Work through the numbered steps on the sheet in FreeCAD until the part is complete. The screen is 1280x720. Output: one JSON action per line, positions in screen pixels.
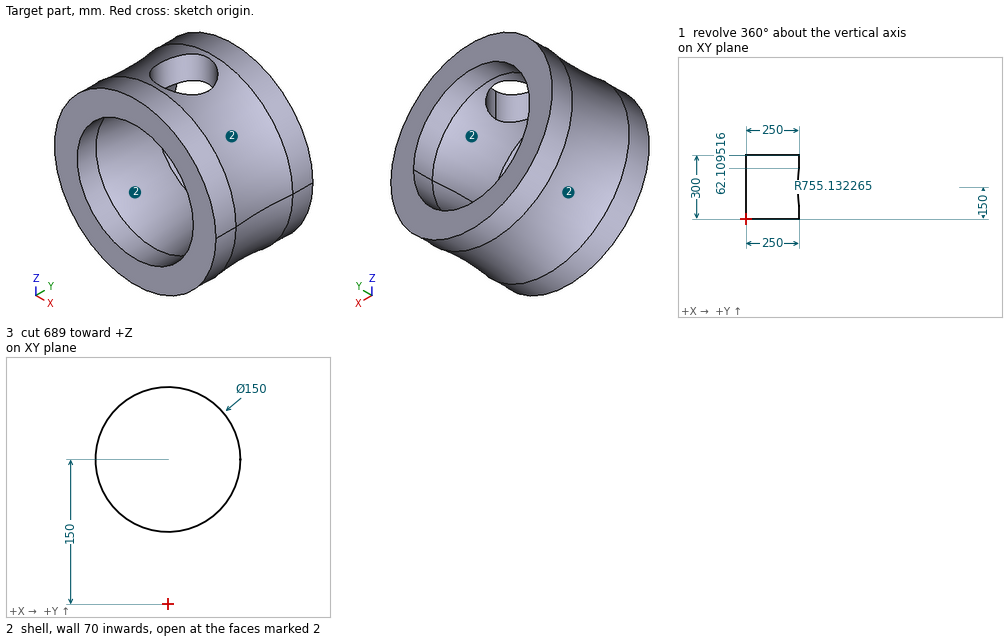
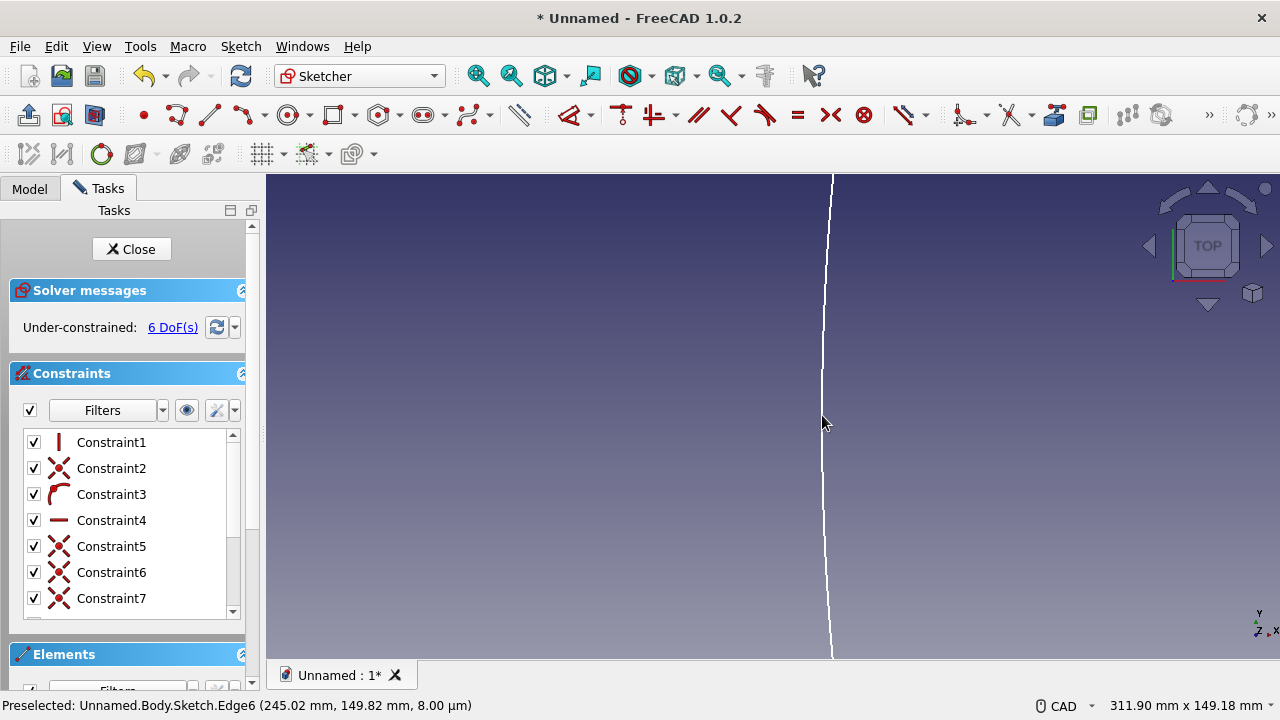
{"action": "left_click", "coordinate": [568, 116]}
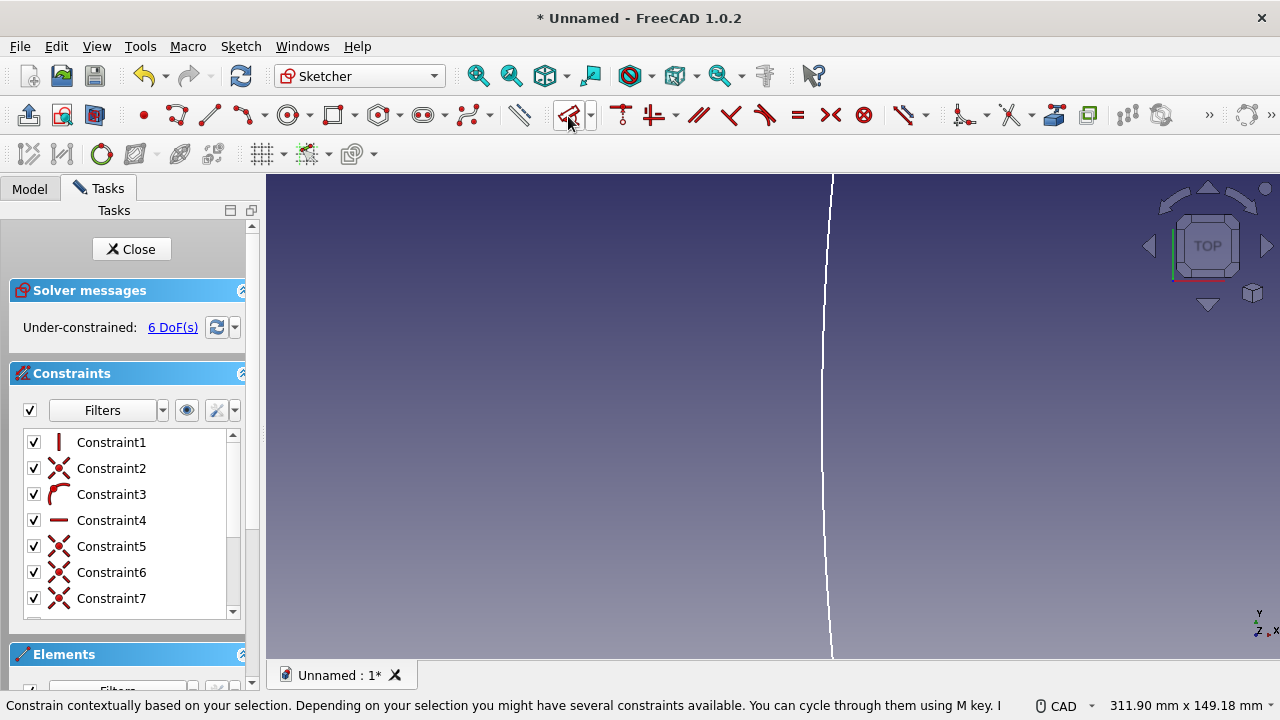
{"action": "left_click", "coordinate": [824, 306]}
{"action": "left_click", "coordinate": [792, 305]}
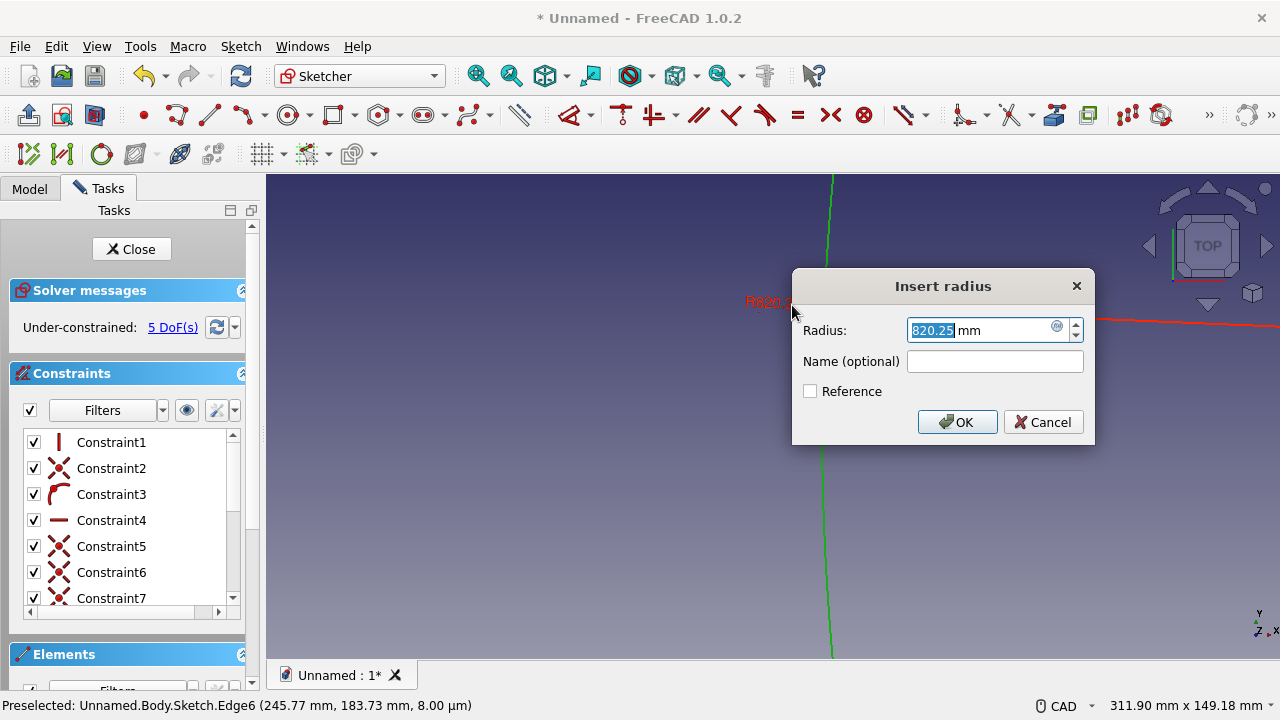
{"action": "type", "text": "755.132265"}
{"action": "key", "text": "Return"}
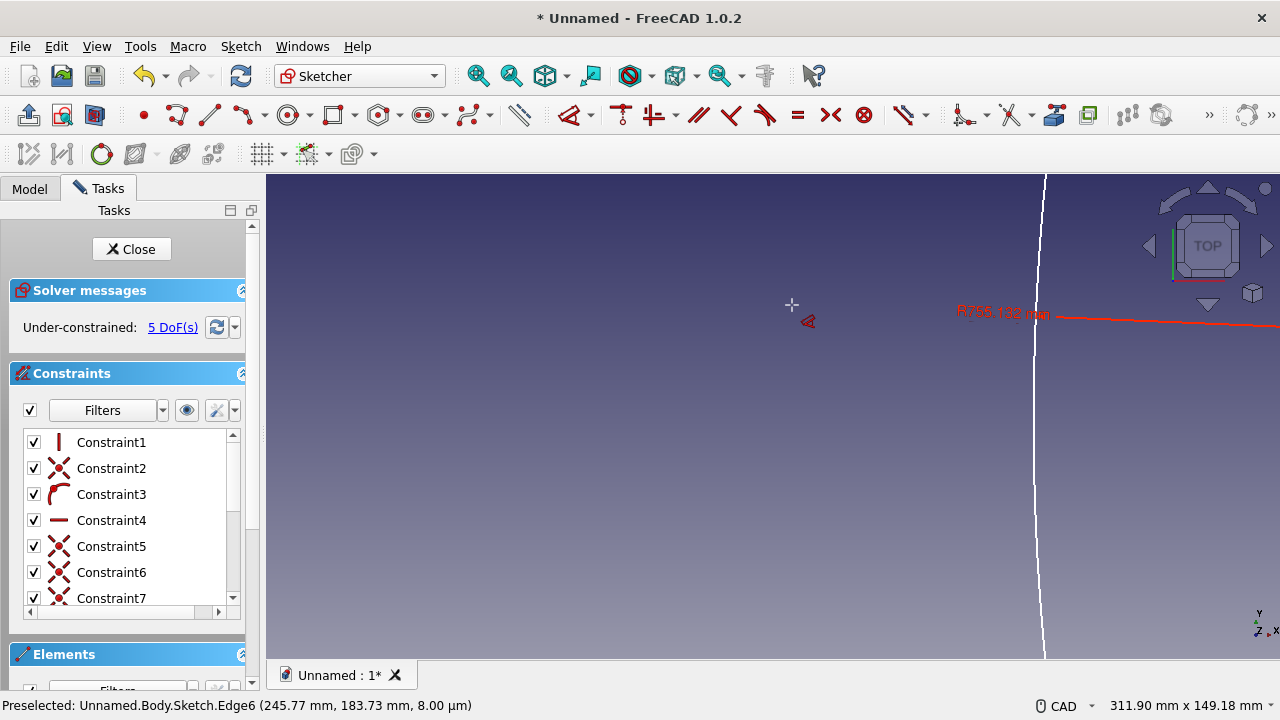
{"action": "scroll", "coordinate": [822, 417], "scroll_direction": "down", "scroll_amount": 6}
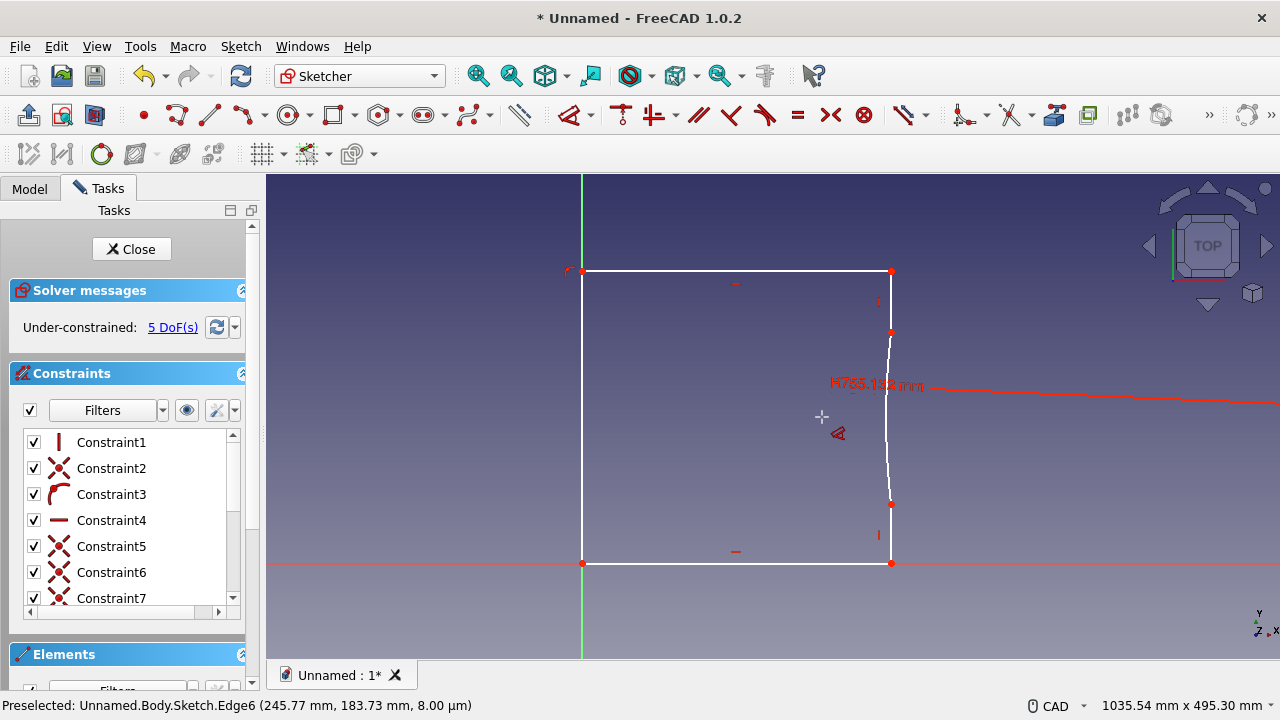
{"action": "left_click", "coordinate": [799, 271]}
{"action": "left_click", "coordinate": [737, 237]}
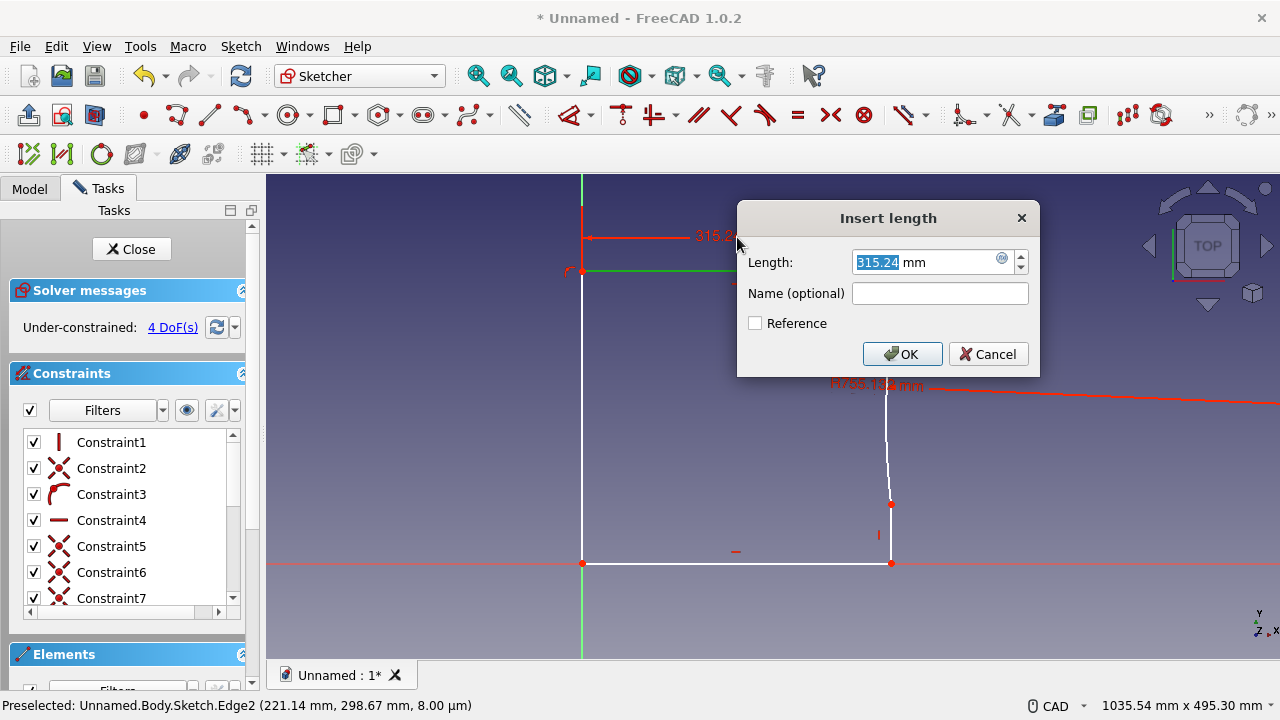
{"action": "type", "text": "250"}
{"action": "key", "text": "Return"}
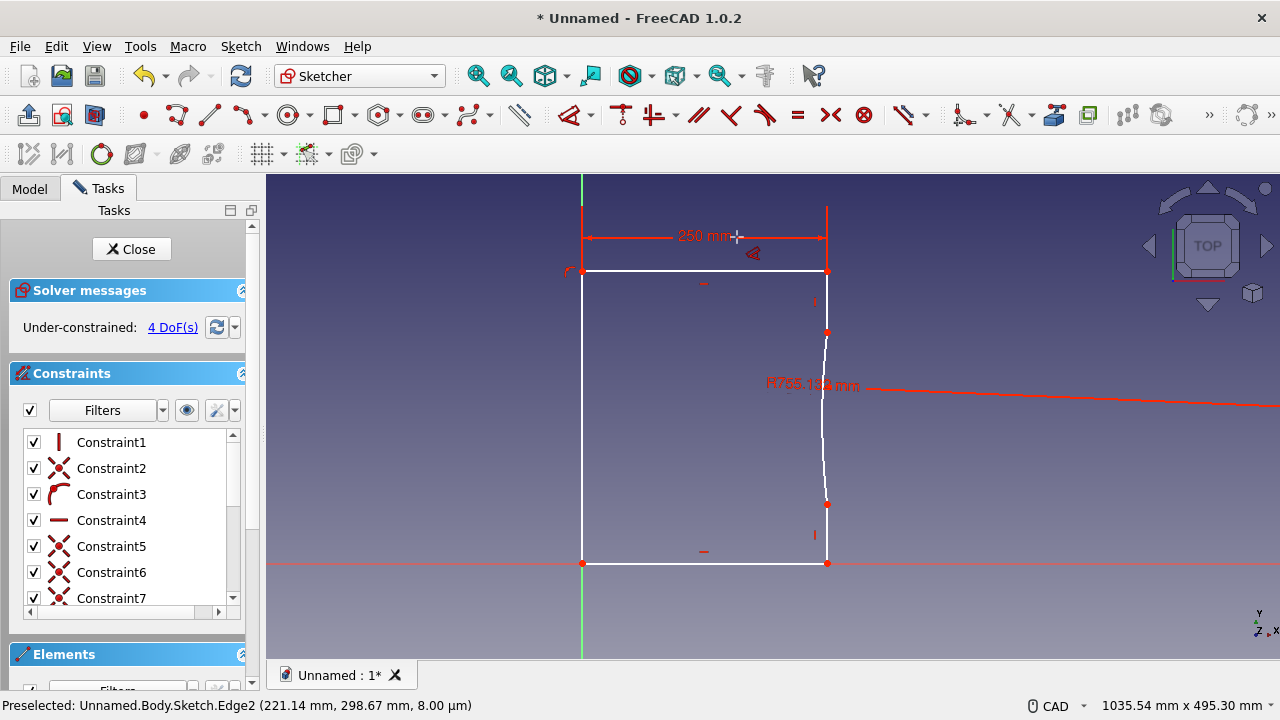
{"action": "left_click", "coordinate": [582, 359]}
{"action": "left_click", "coordinate": [548, 418]}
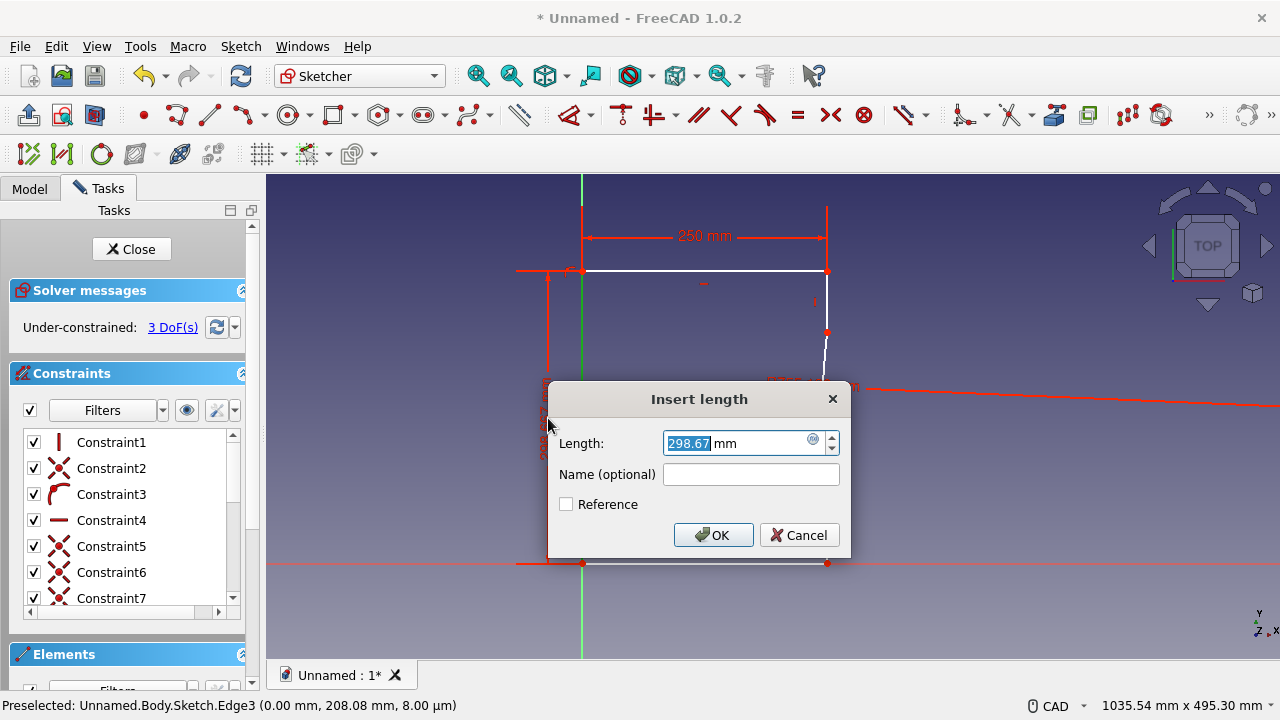
{"action": "type", "text": "300"}
{"action": "key", "text": "Return"}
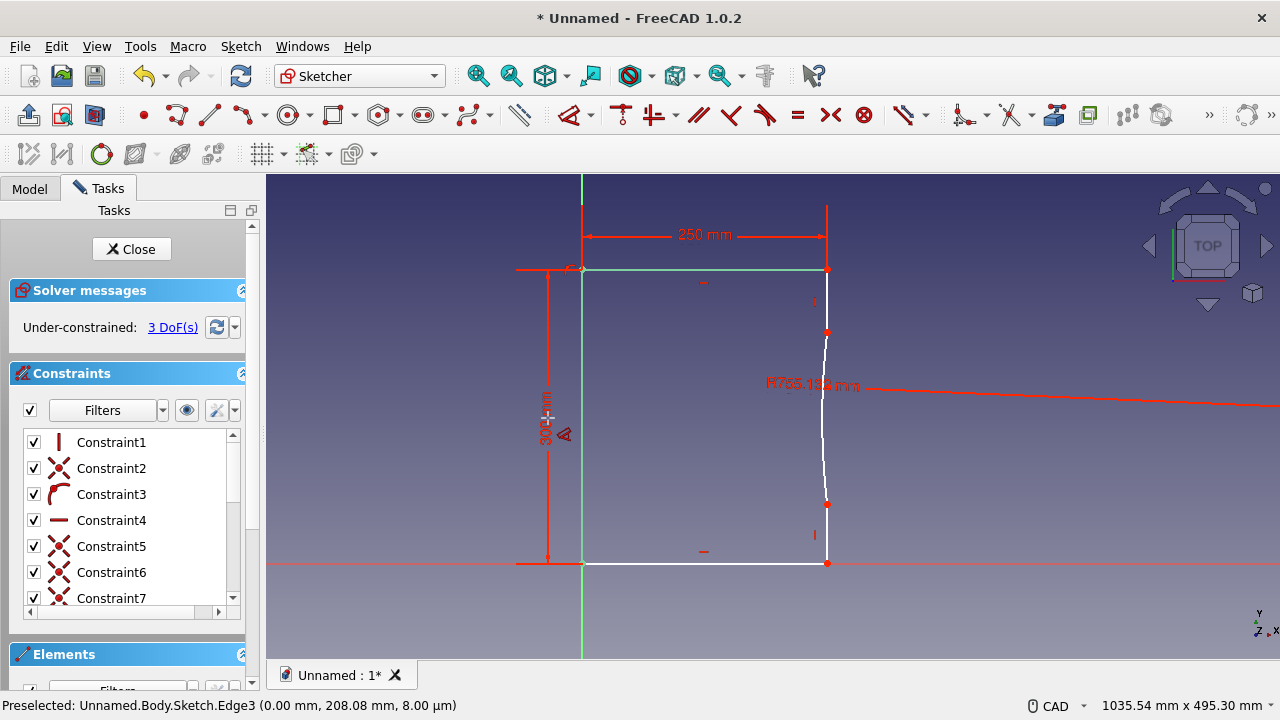
{"action": "left_click", "coordinate": [827, 564]}
{"action": "left_click", "coordinate": [705, 598]}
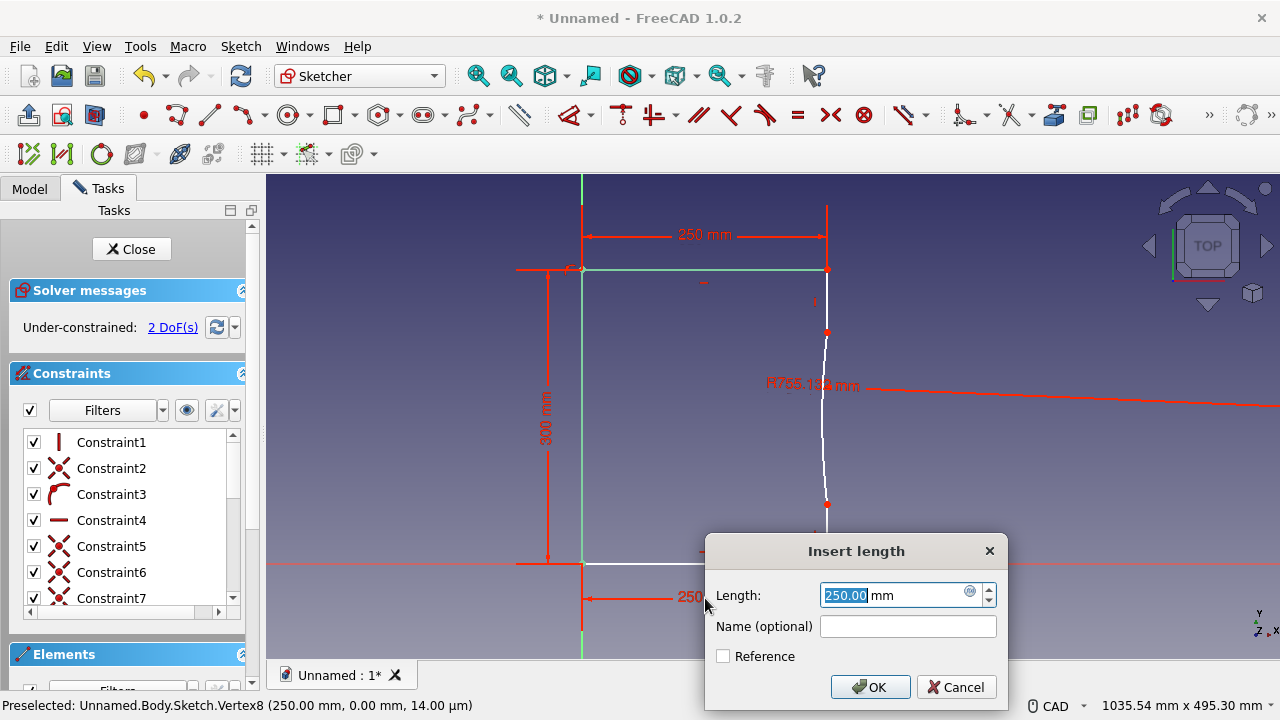
{"action": "type", "text": "250"}
{"action": "key", "text": "Return"}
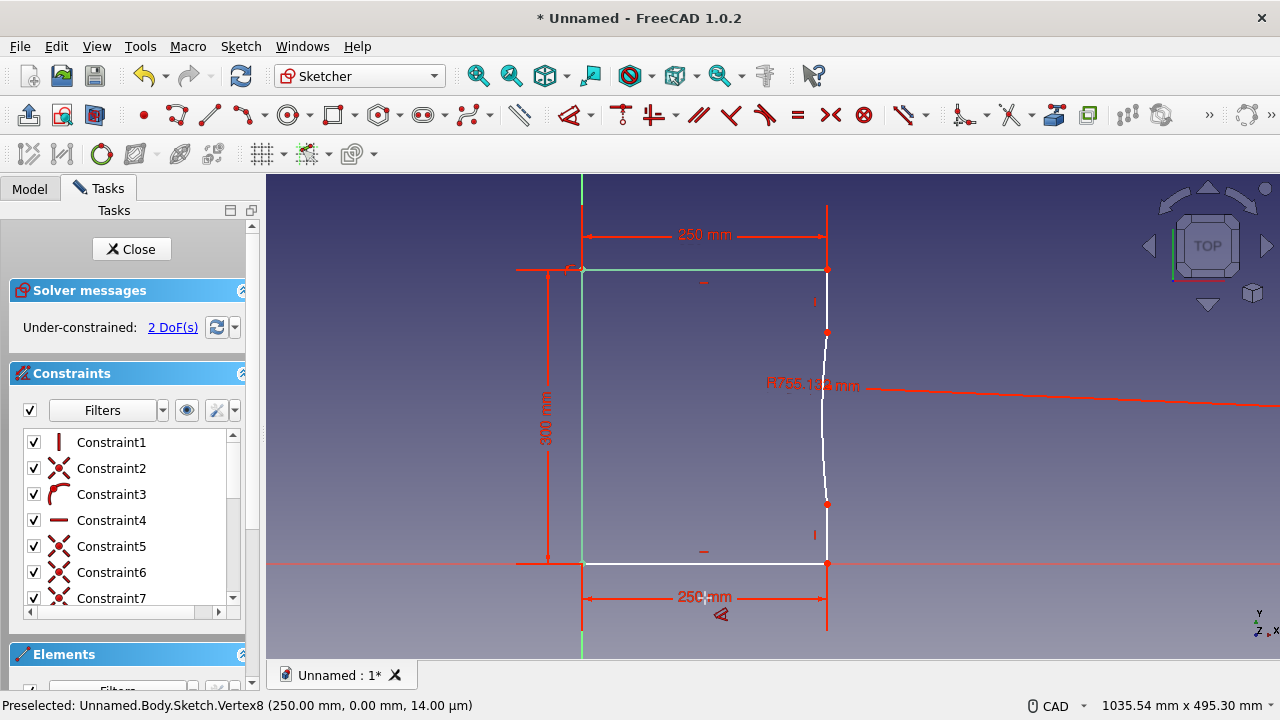
{"action": "scroll", "coordinate": [294, 416], "scroll_direction": "down", "scroll_amount": 3}